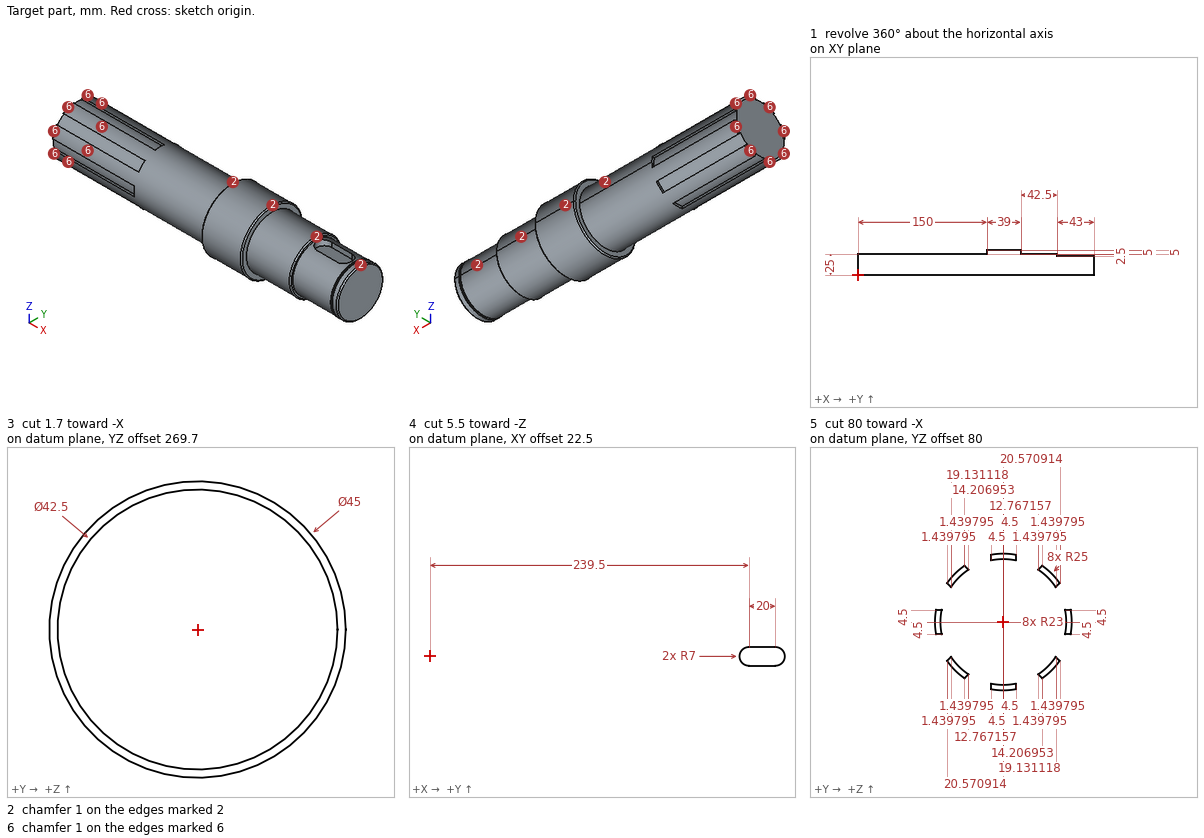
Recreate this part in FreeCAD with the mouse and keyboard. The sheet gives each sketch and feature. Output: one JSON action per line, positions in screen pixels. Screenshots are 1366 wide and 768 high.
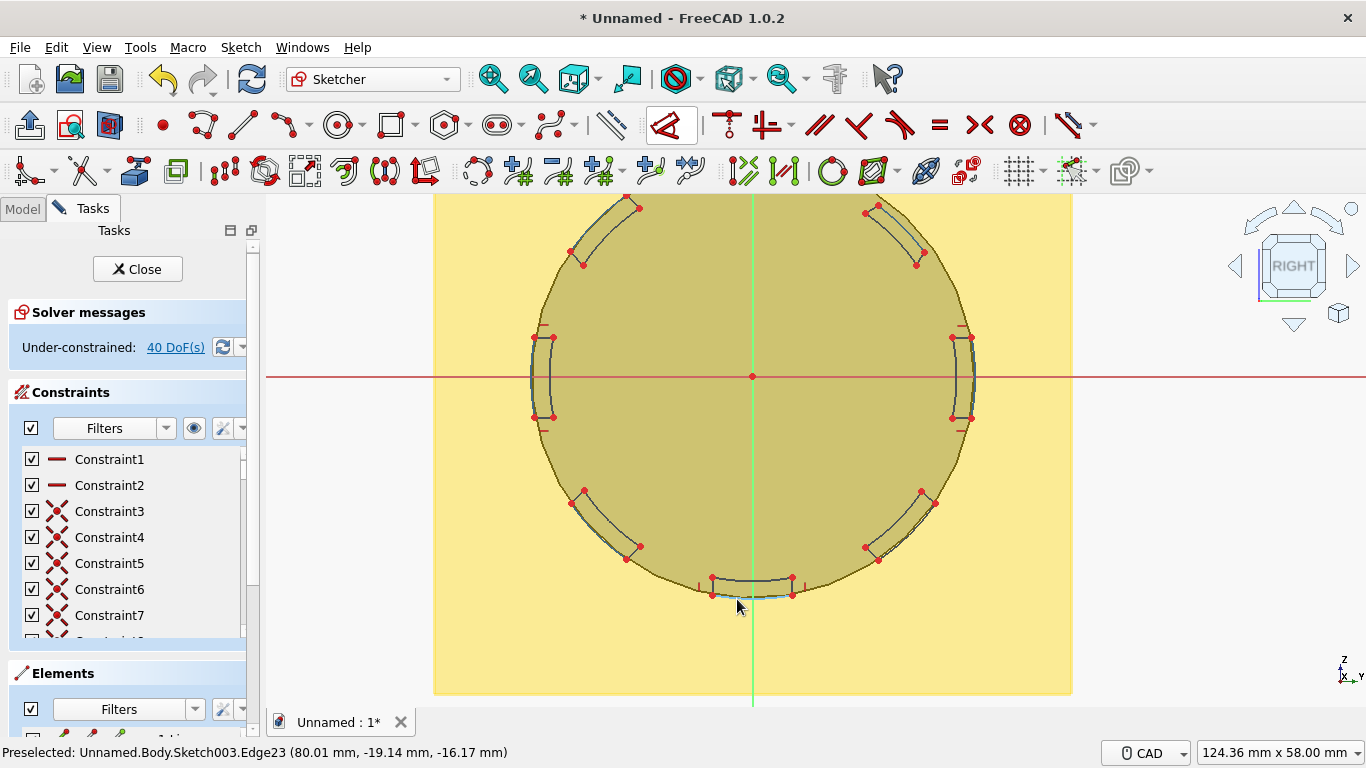
{"action": "left_click", "coordinate": [736, 598]}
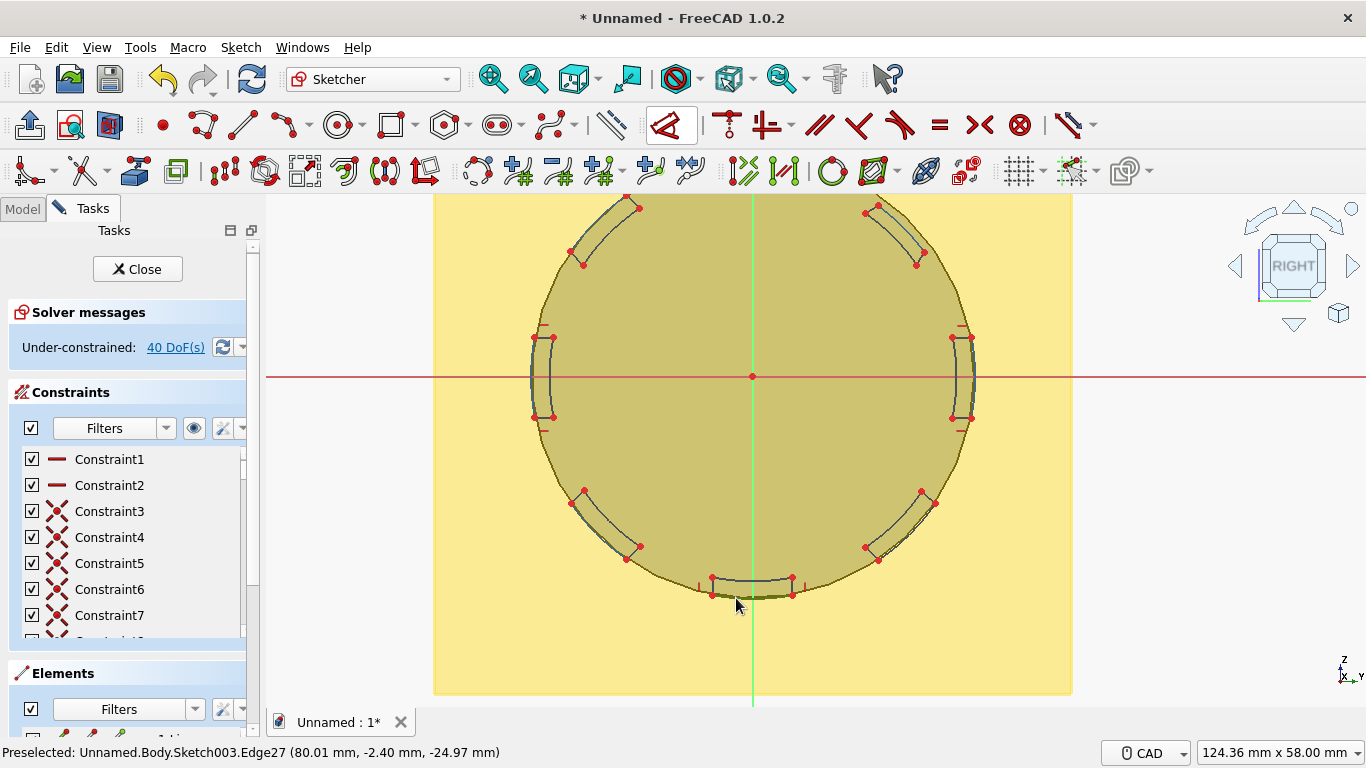
{"action": "left_click", "coordinate": [898, 546]}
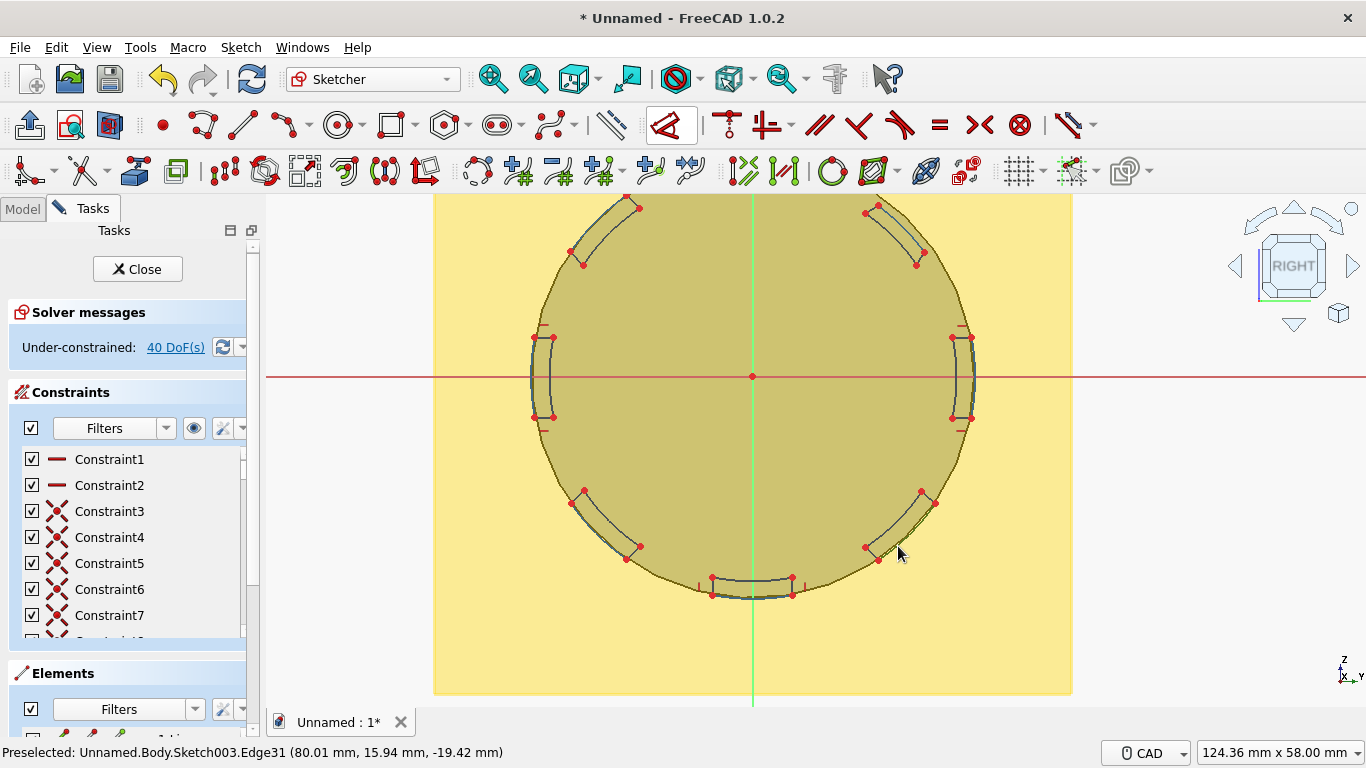
{"action": "left_click", "coordinate": [940, 126]}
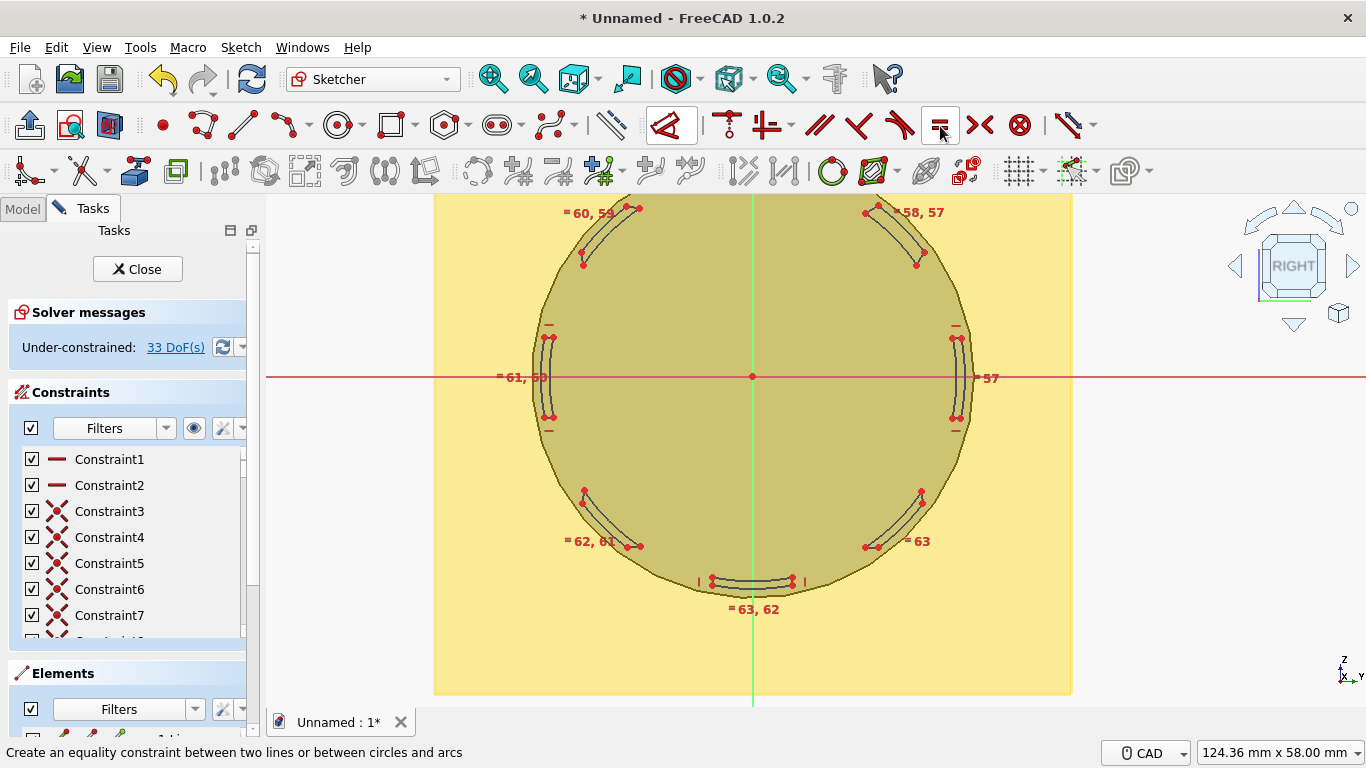
{"action": "scroll", "coordinate": [956, 362], "scroll_direction": "up", "scroll_amount": 3}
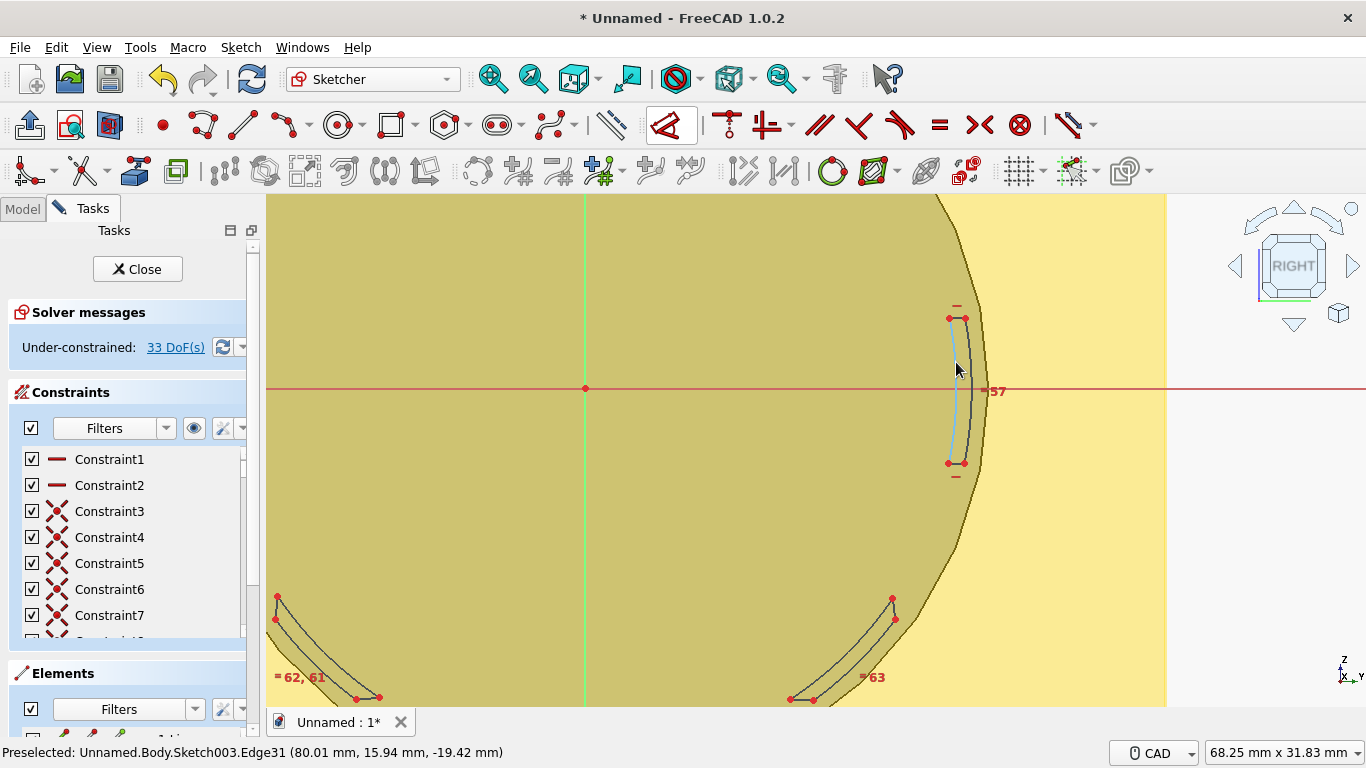
{"action": "left_click", "coordinate": [955, 362]}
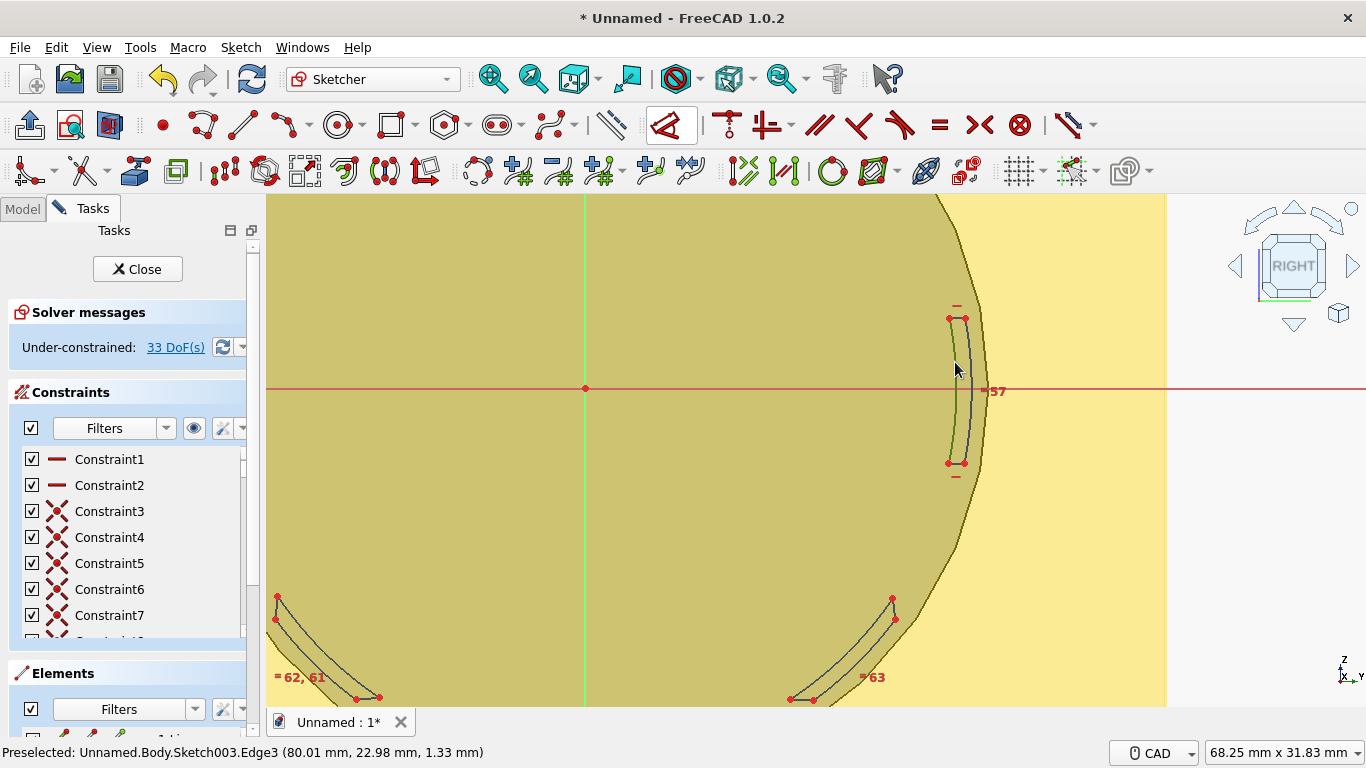
{"action": "scroll", "coordinate": [842, 486], "scroll_direction": "down", "scroll_amount": 5}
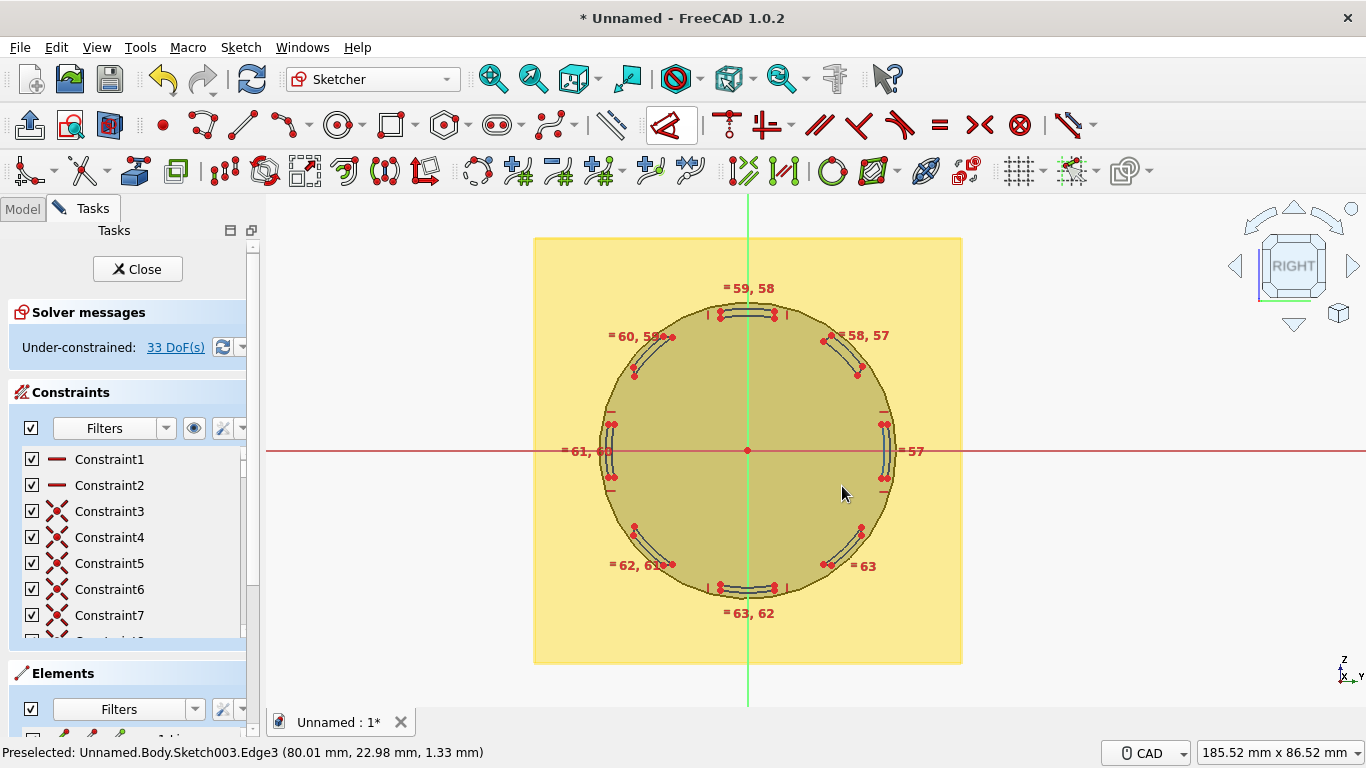
{"action": "scroll", "coordinate": [849, 364], "scroll_direction": "up", "scroll_amount": 3}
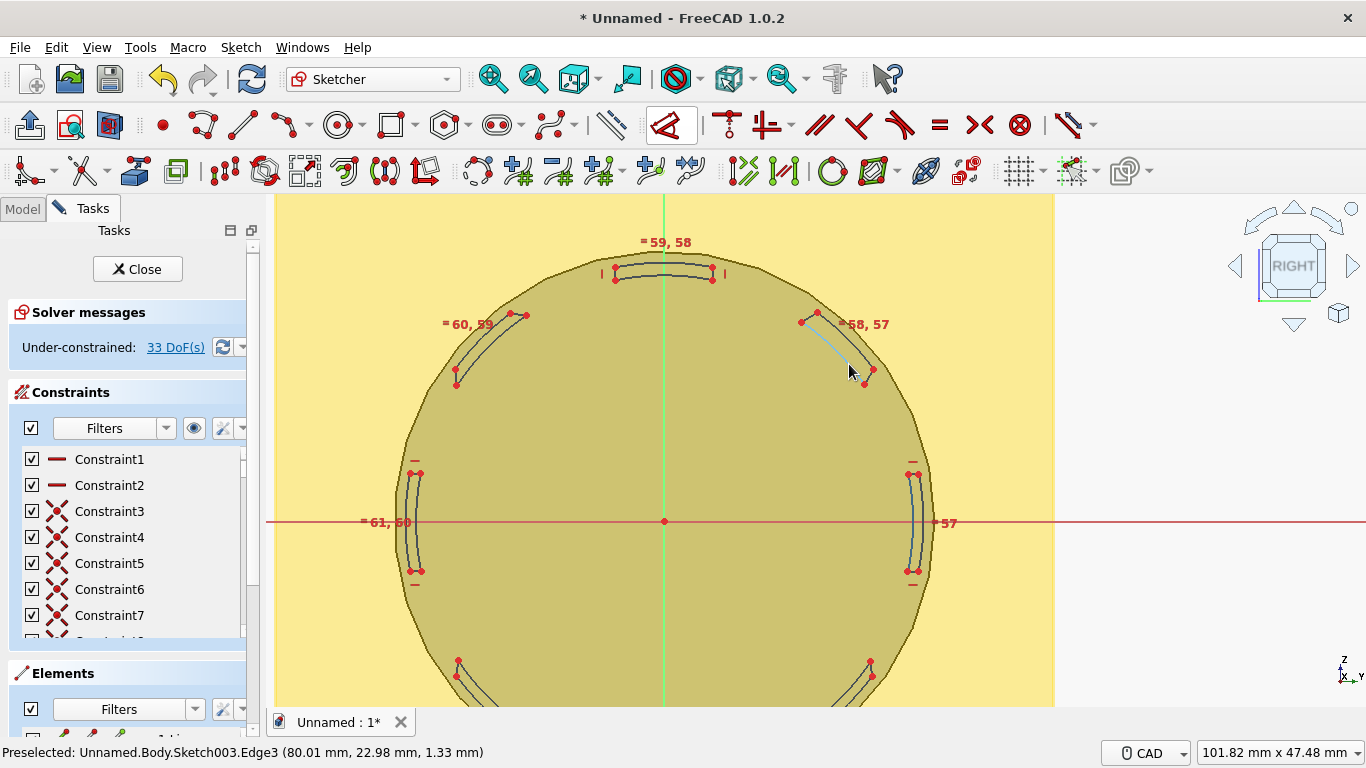
{"action": "left_click", "coordinate": [848, 364]}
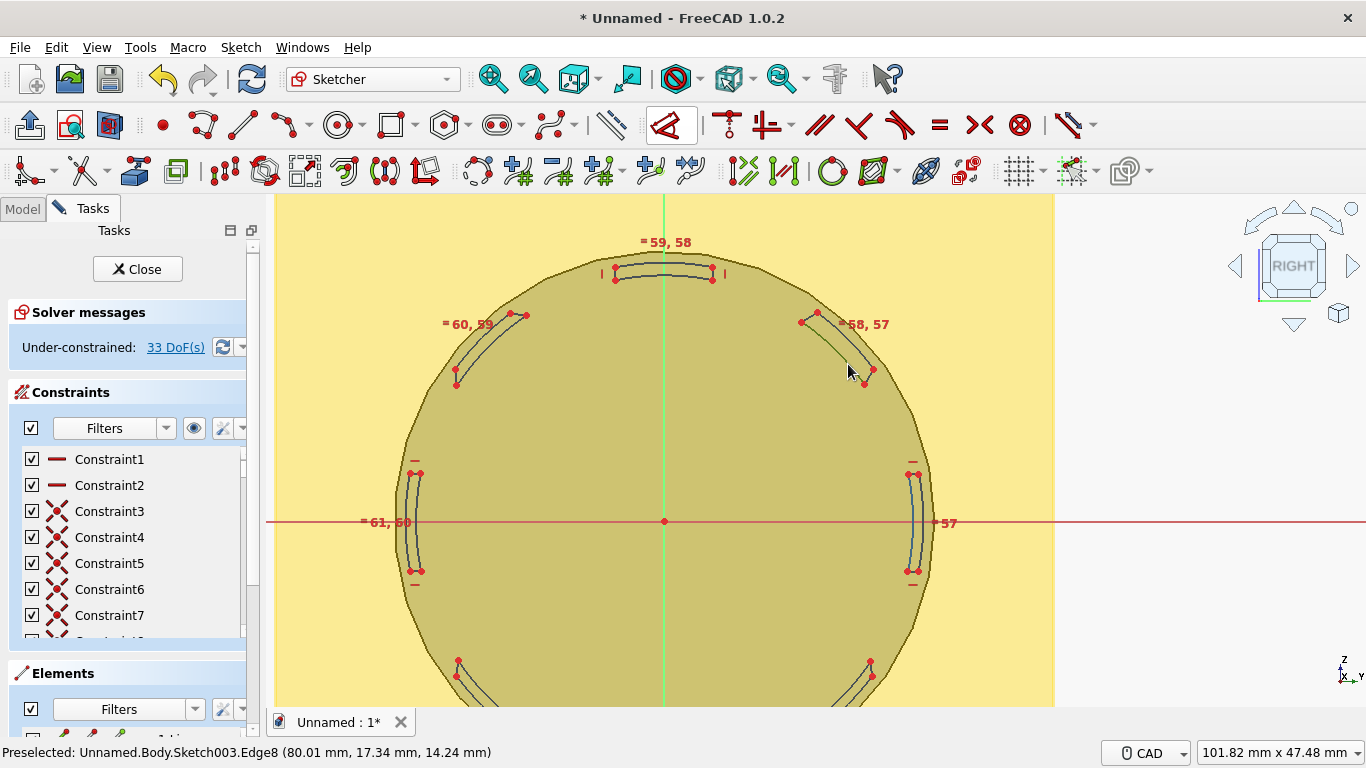
{"action": "left_click", "coordinate": [684, 276]}